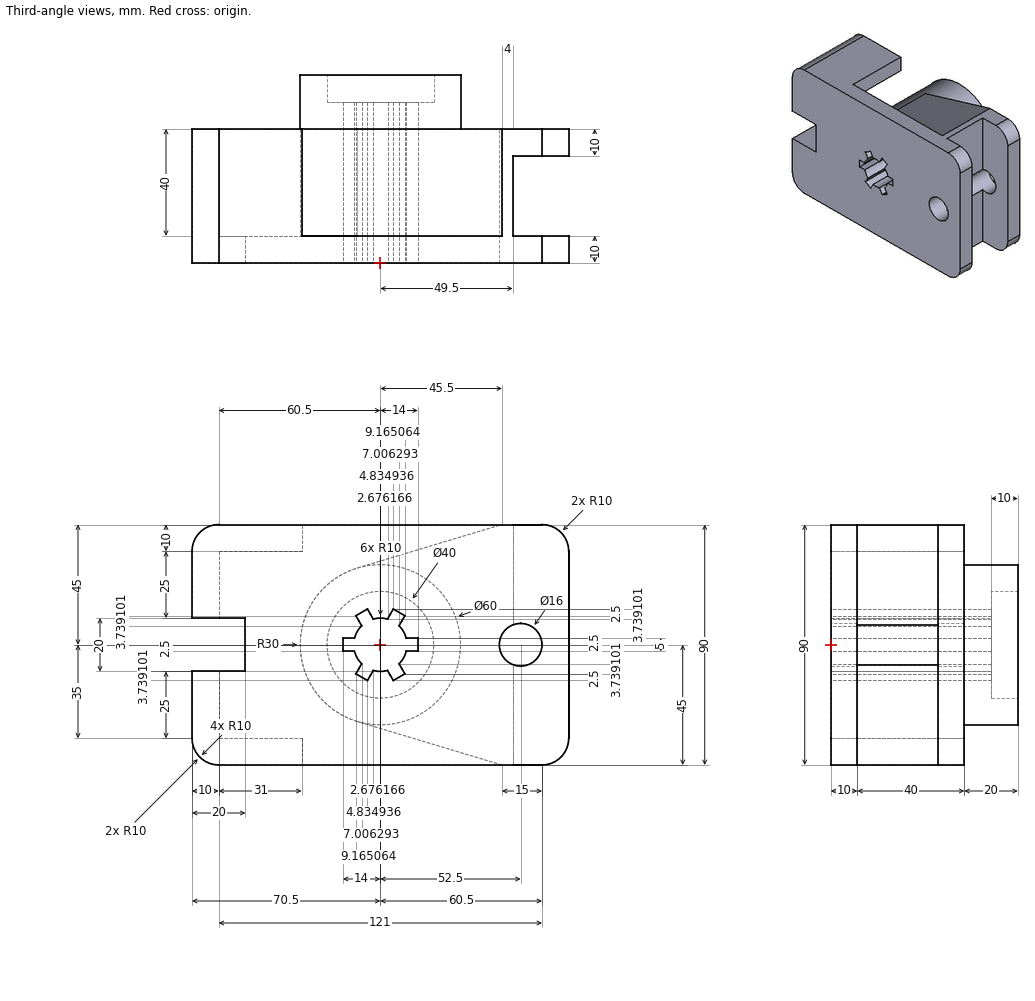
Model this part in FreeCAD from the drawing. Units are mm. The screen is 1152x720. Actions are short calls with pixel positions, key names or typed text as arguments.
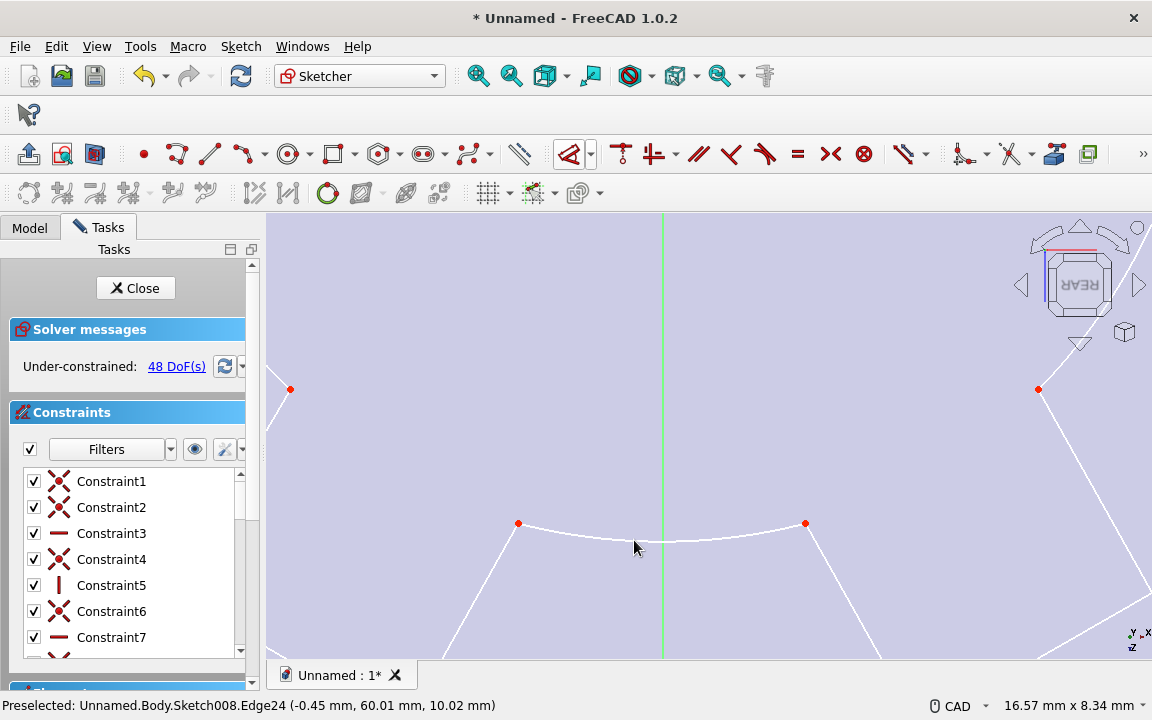
scroll(635, 545, down, 8)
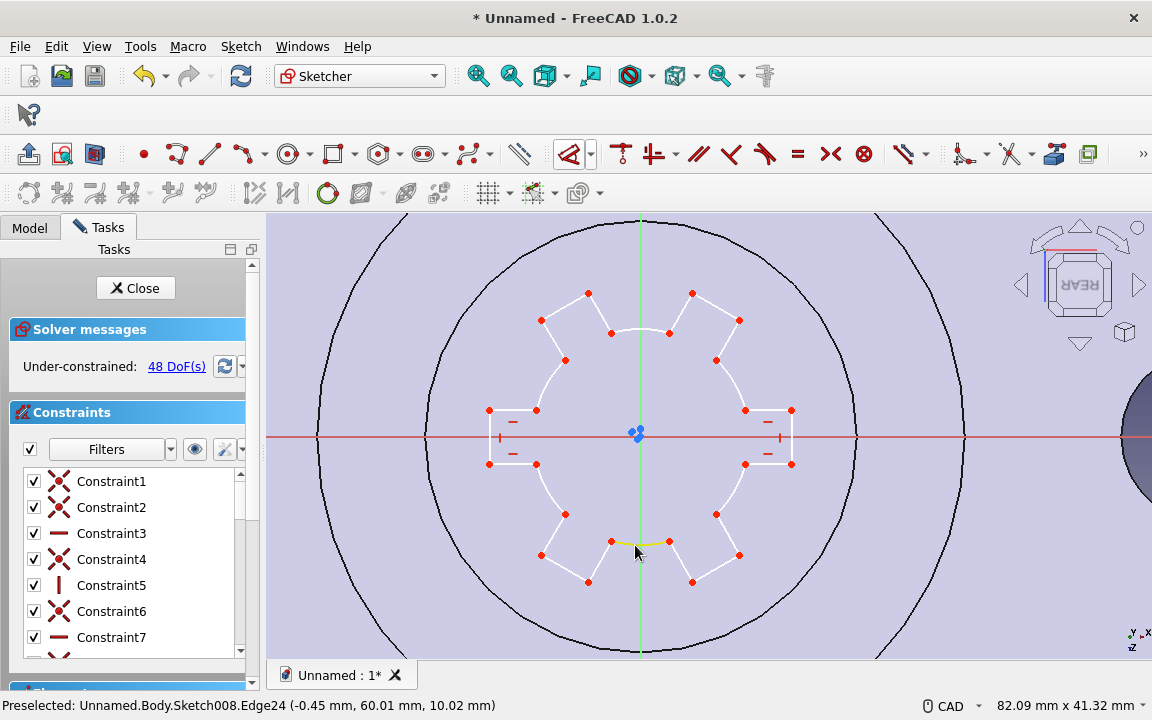
click(728, 501)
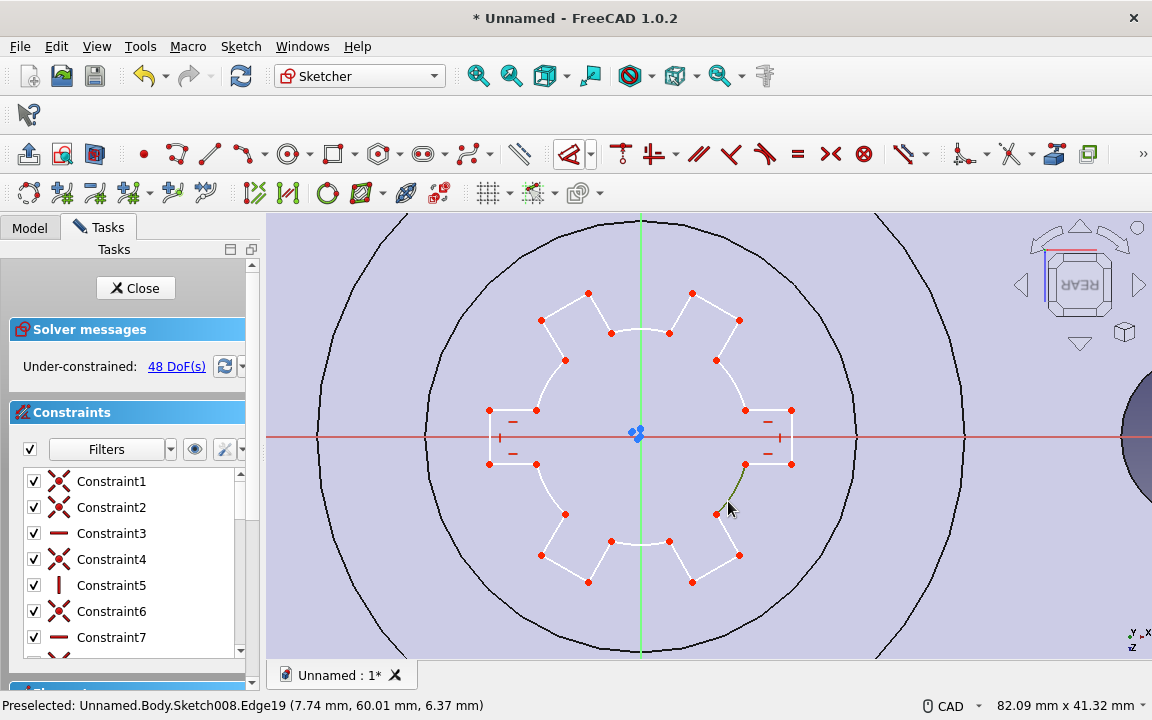
click(740, 394)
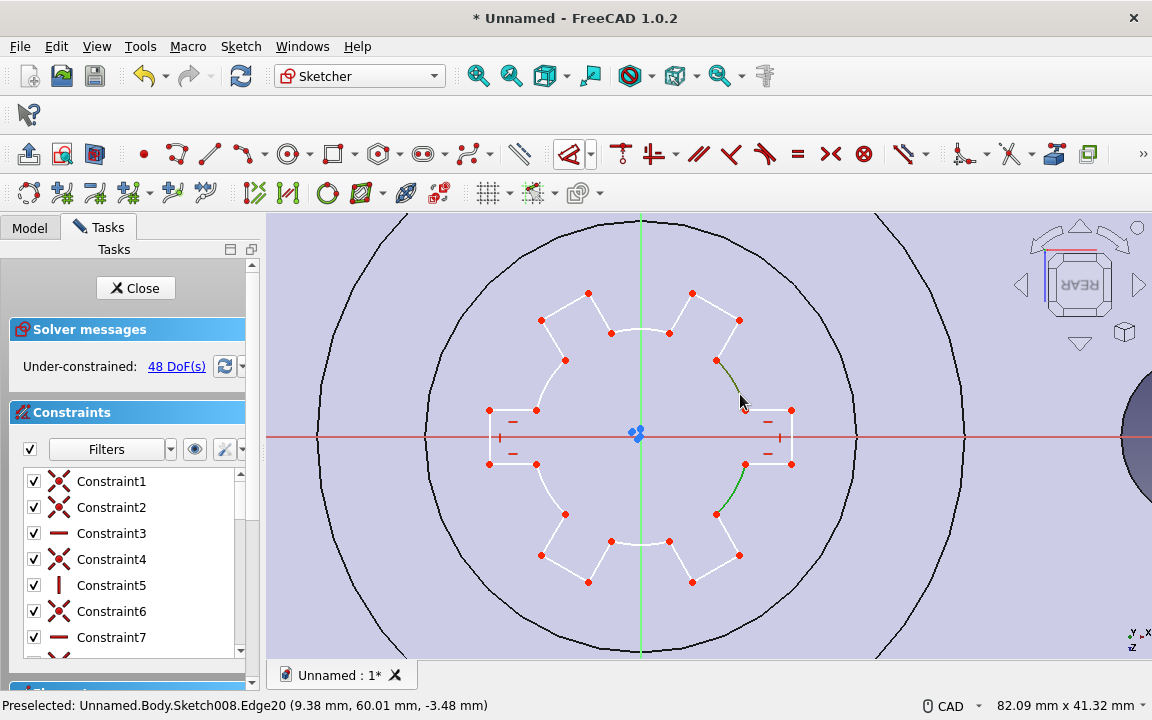
click(621, 154)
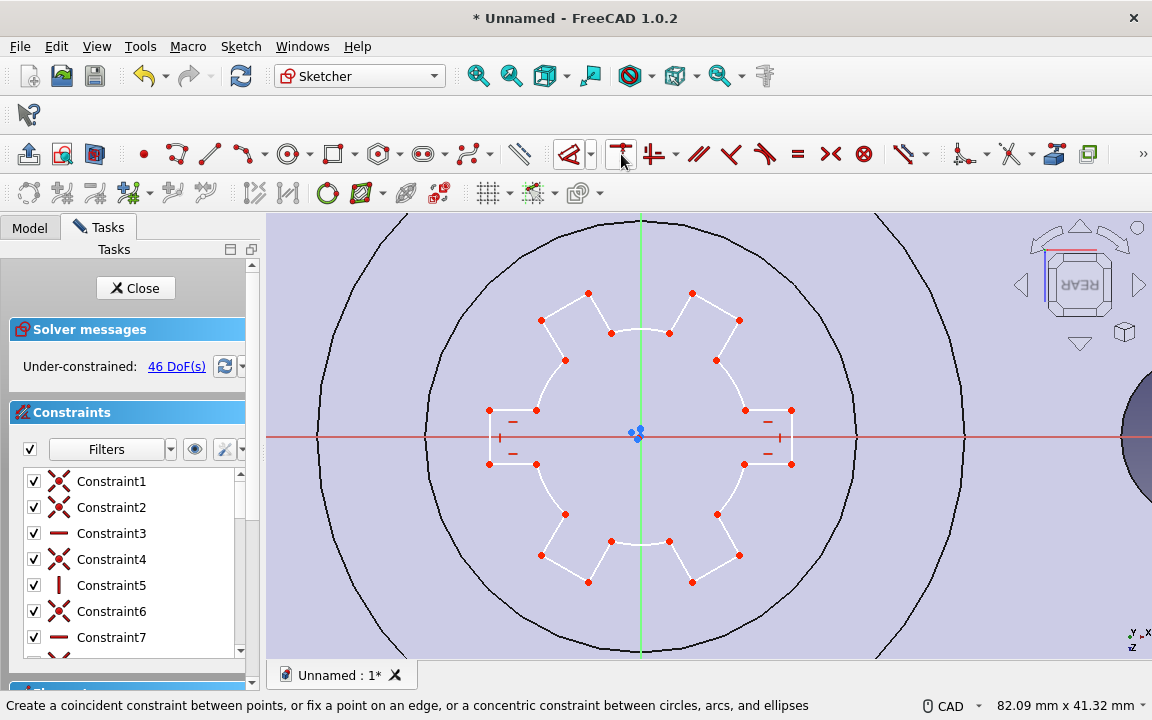
click(728, 501)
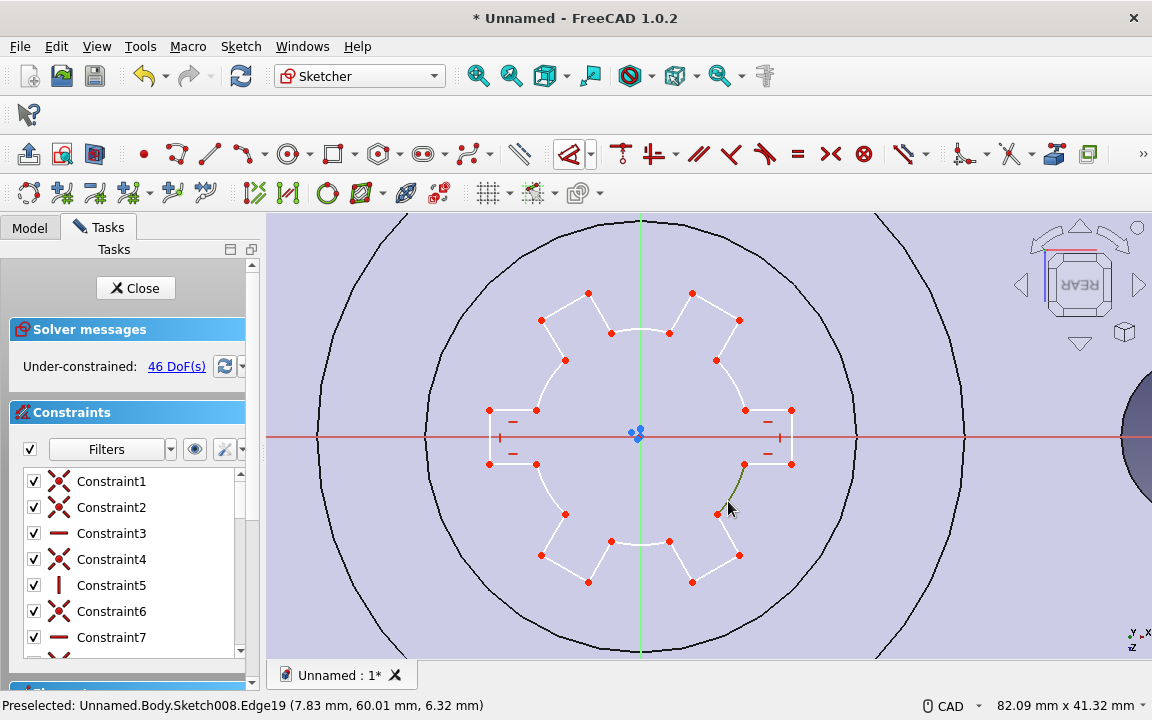
click(652, 330)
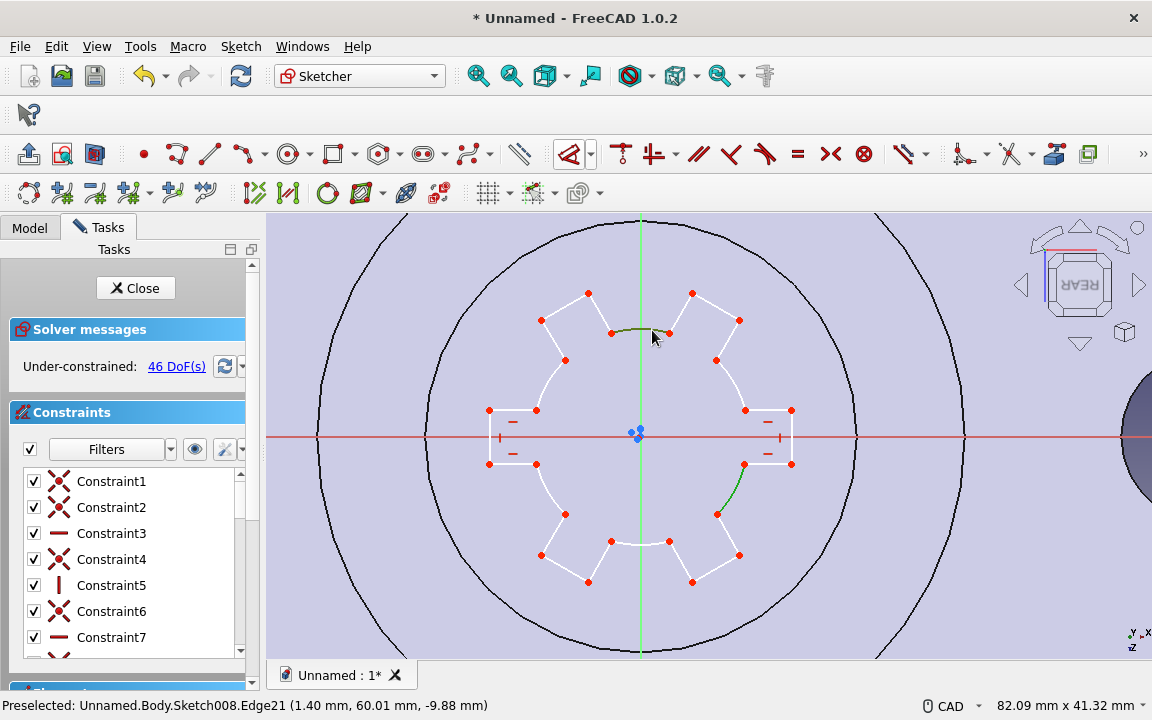
click(621, 154)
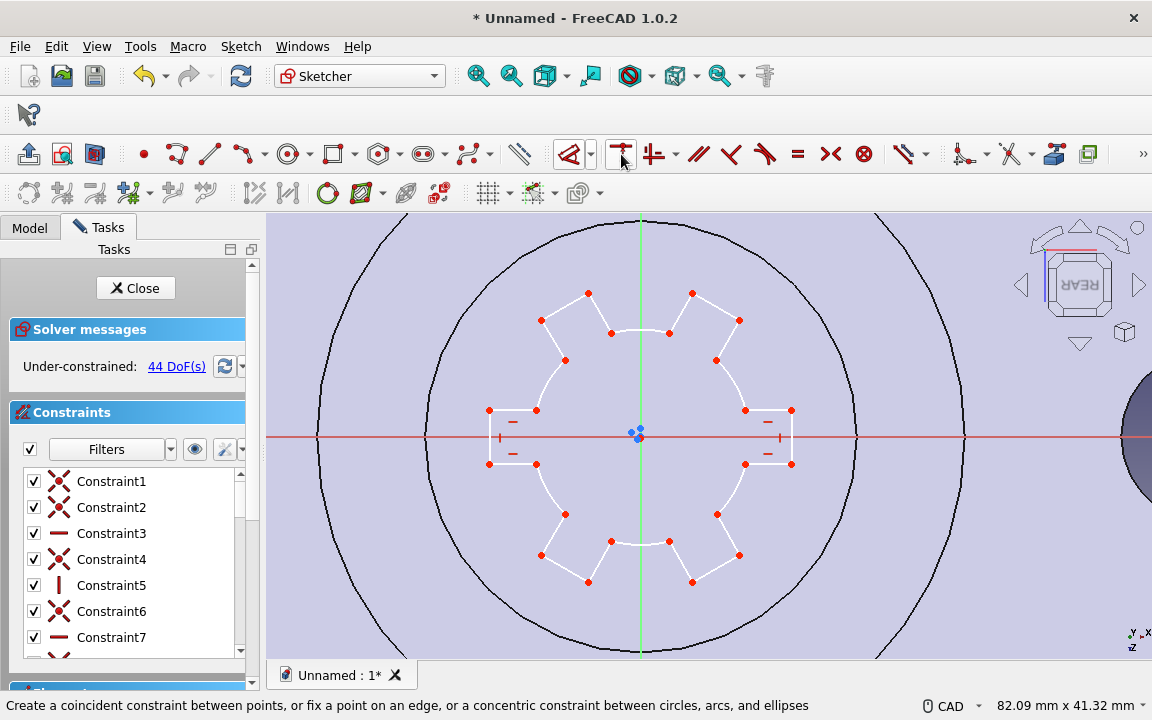
click(728, 501)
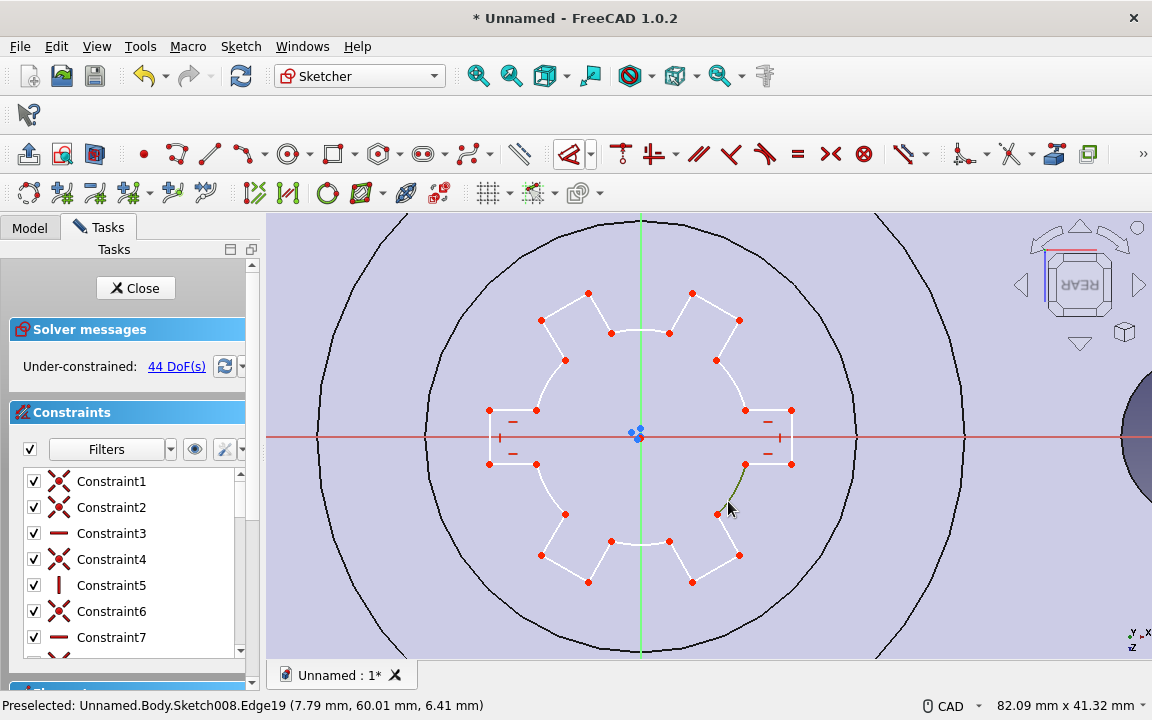
click(554, 373)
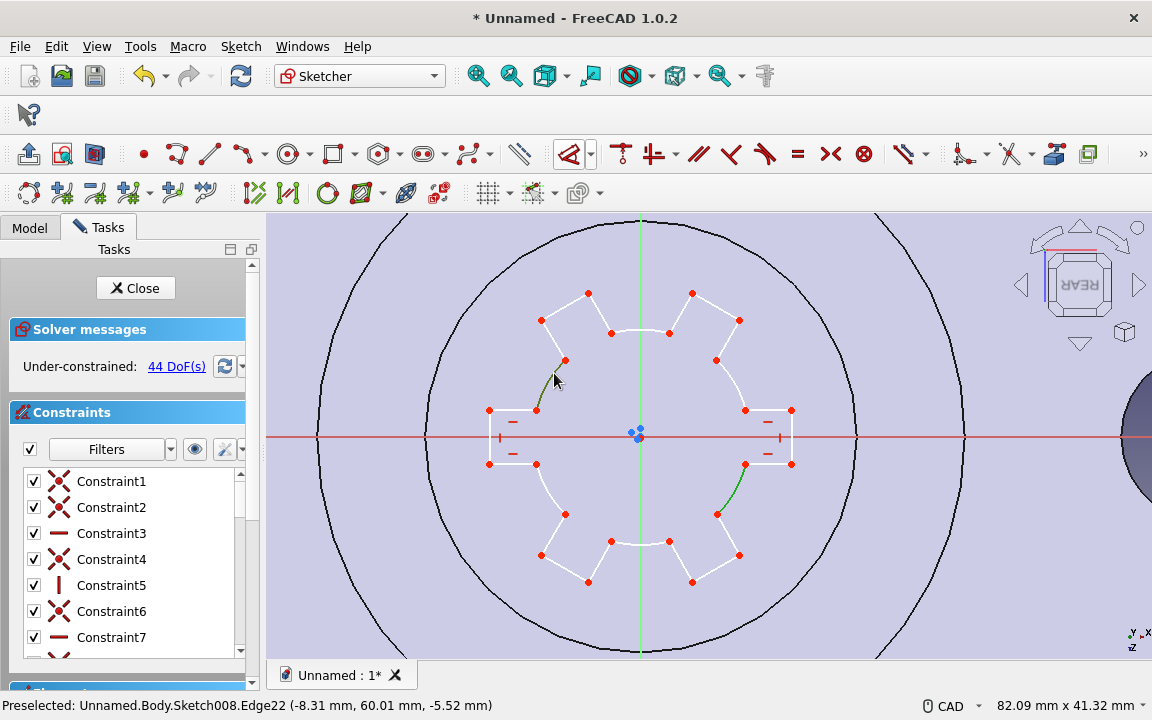
click(621, 154)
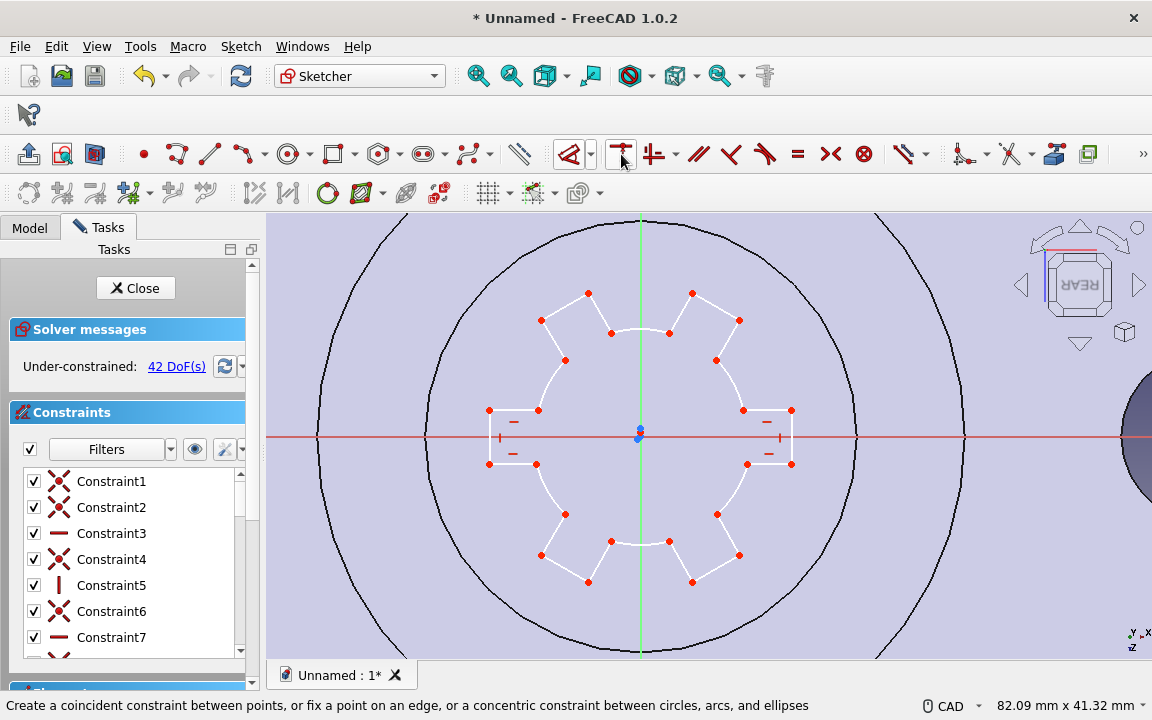
click(729, 501)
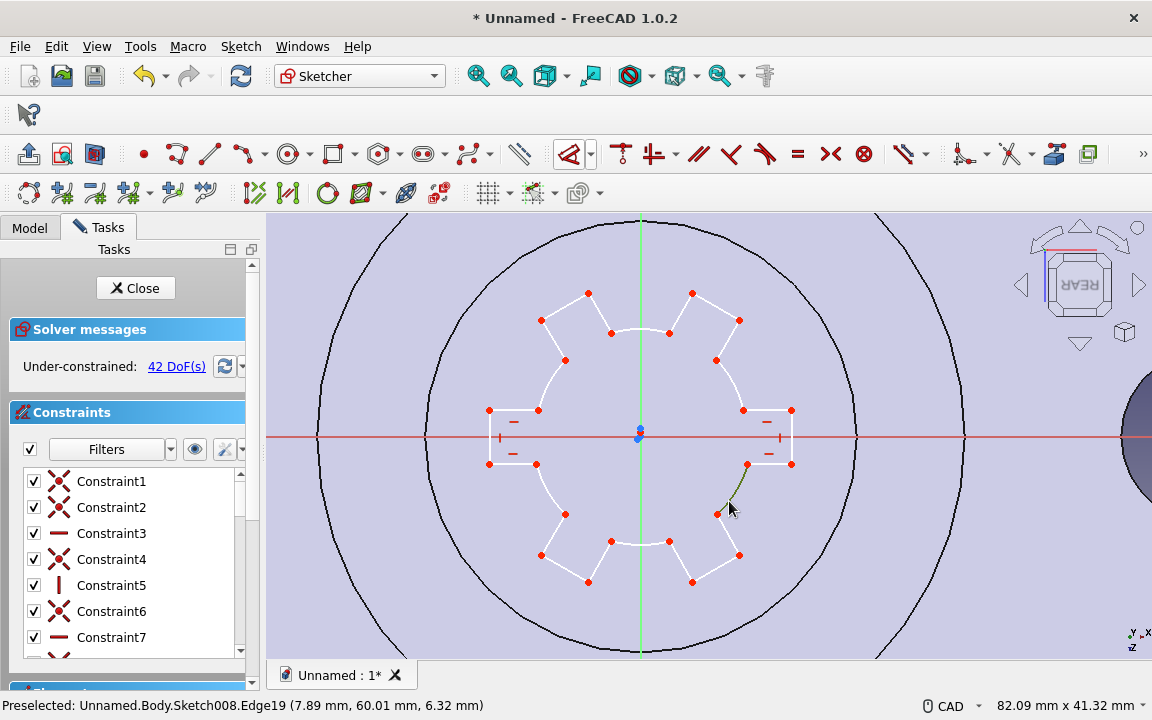
click(542, 481)